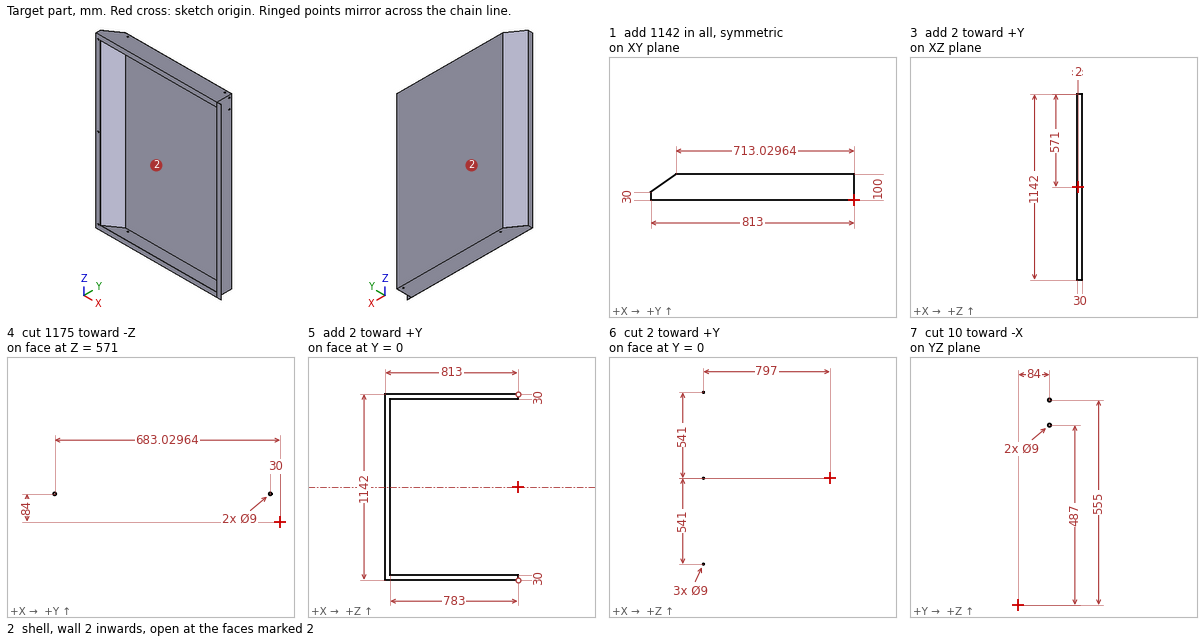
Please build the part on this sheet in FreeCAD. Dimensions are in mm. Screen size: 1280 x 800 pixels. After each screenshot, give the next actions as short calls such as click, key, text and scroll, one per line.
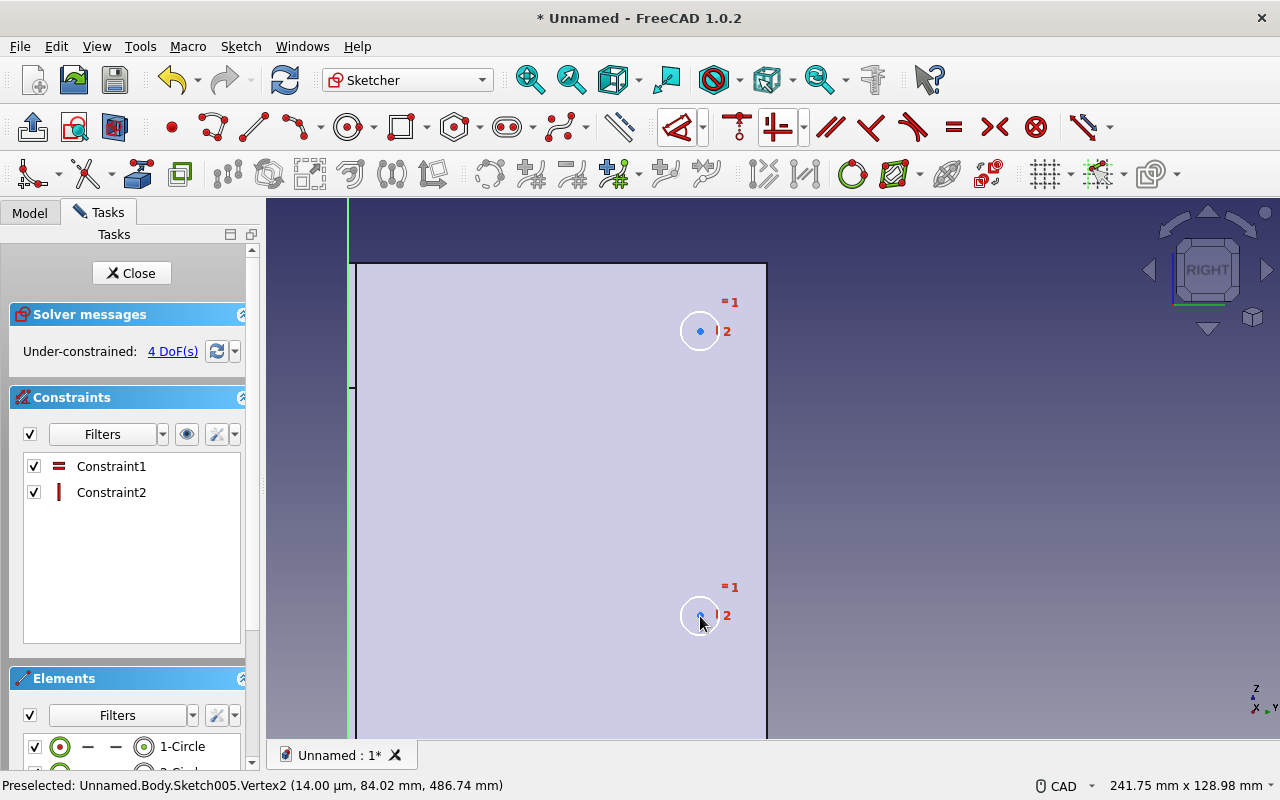
click(713, 317)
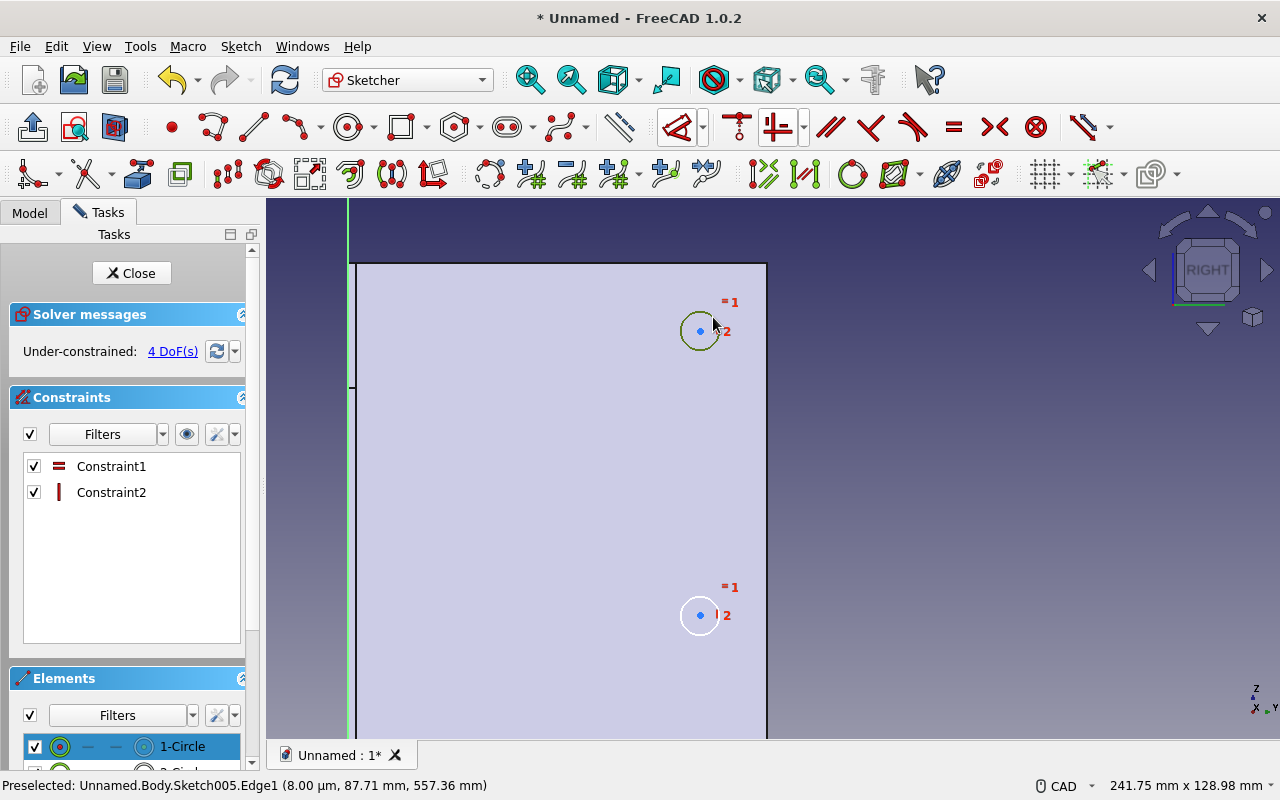
click(702, 128)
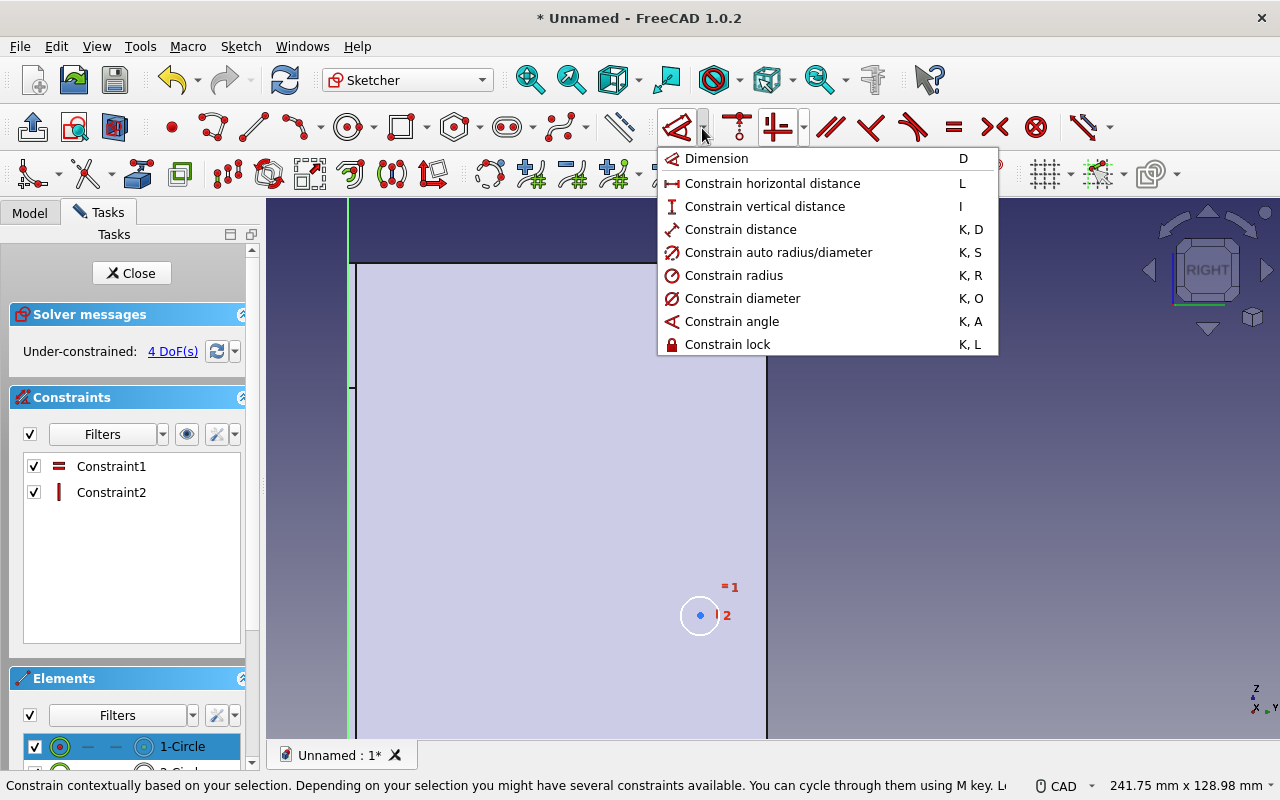
click(828, 298)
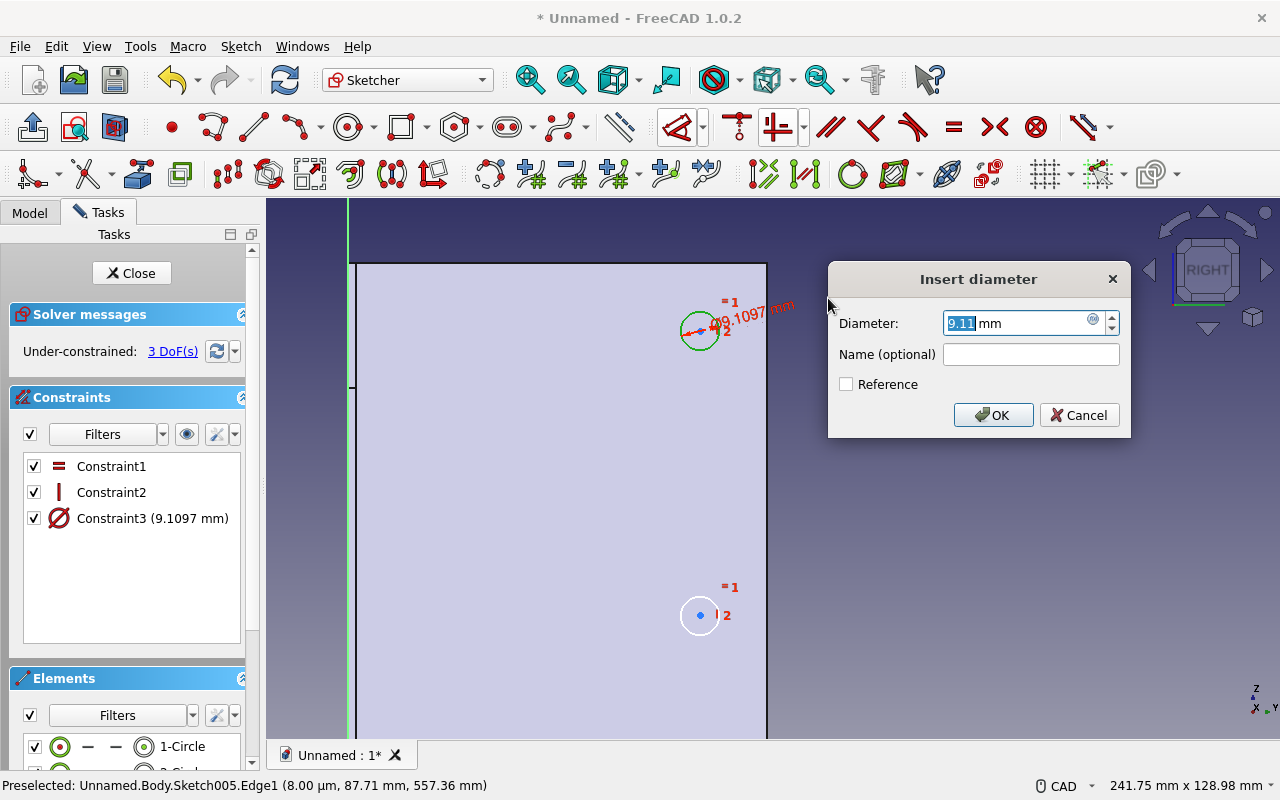
text(9)
key(Return)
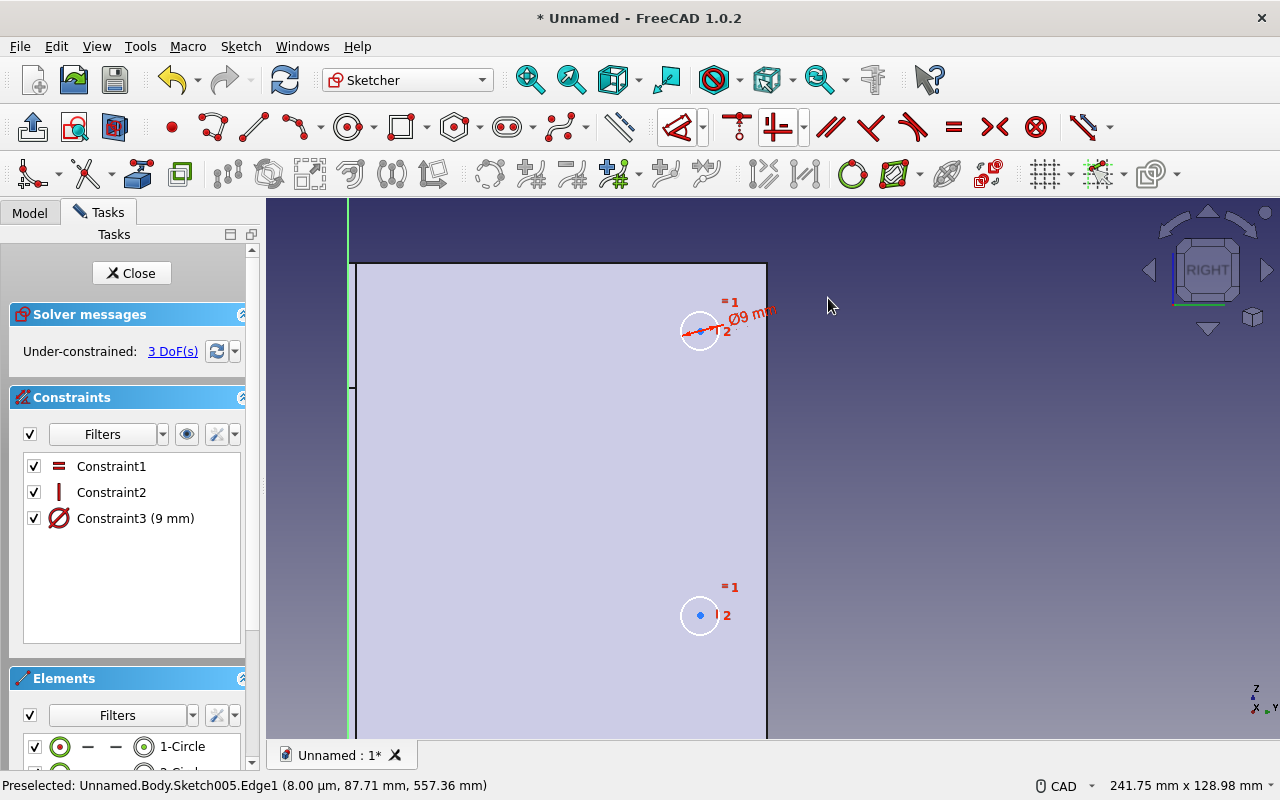
click(700, 331)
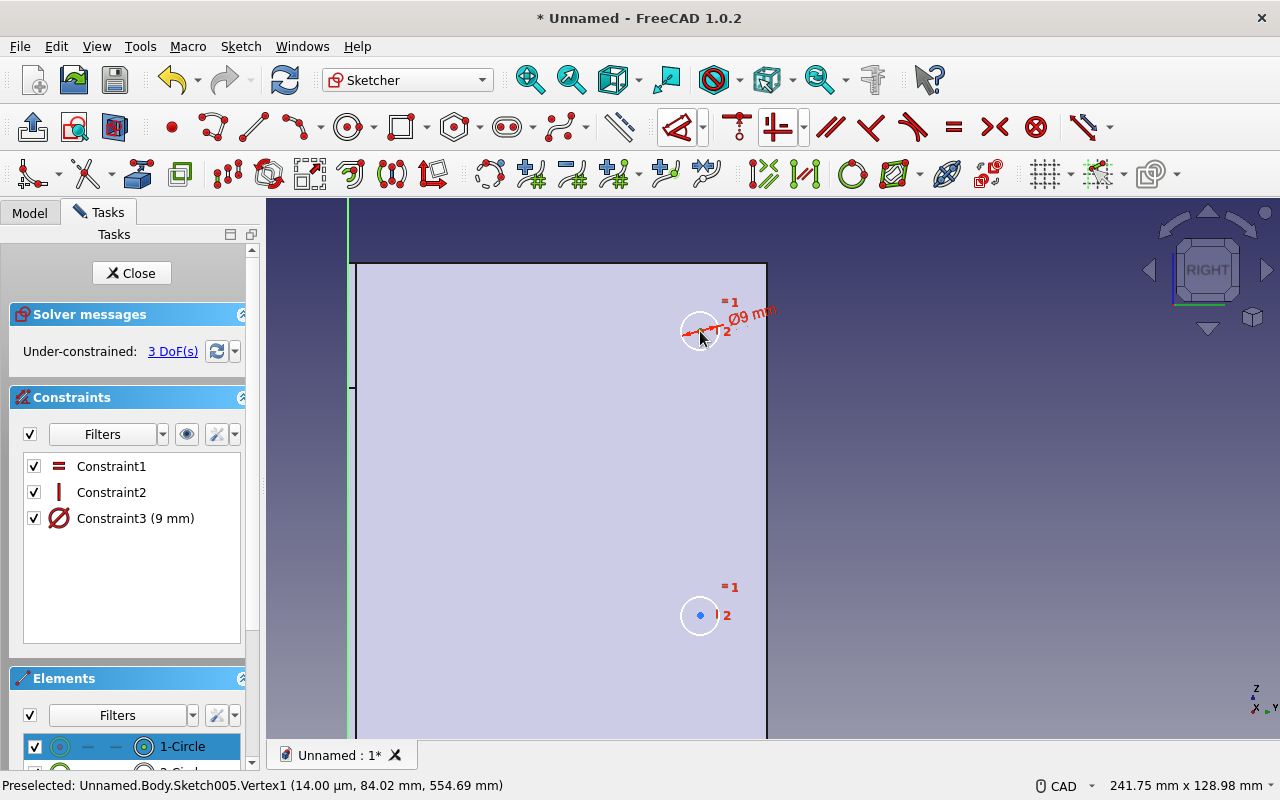
key(l)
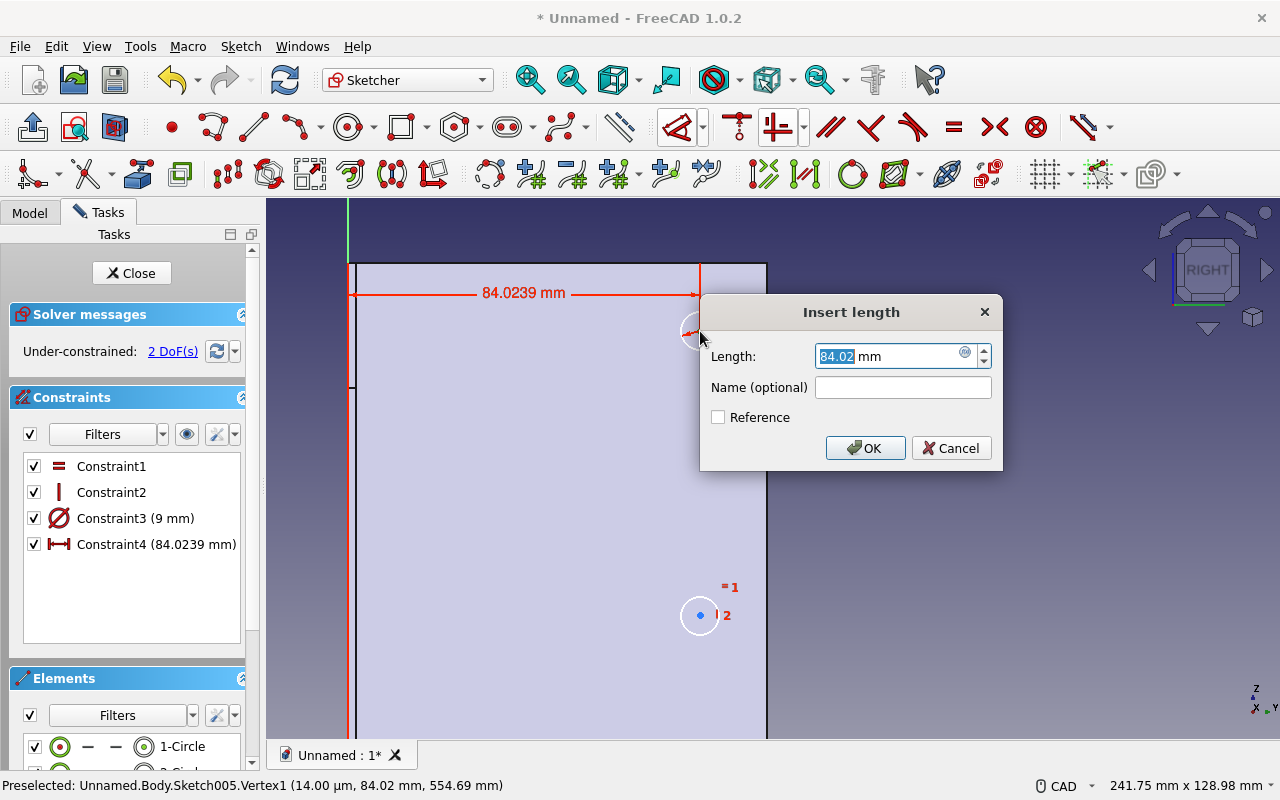
text(84)
key(Return)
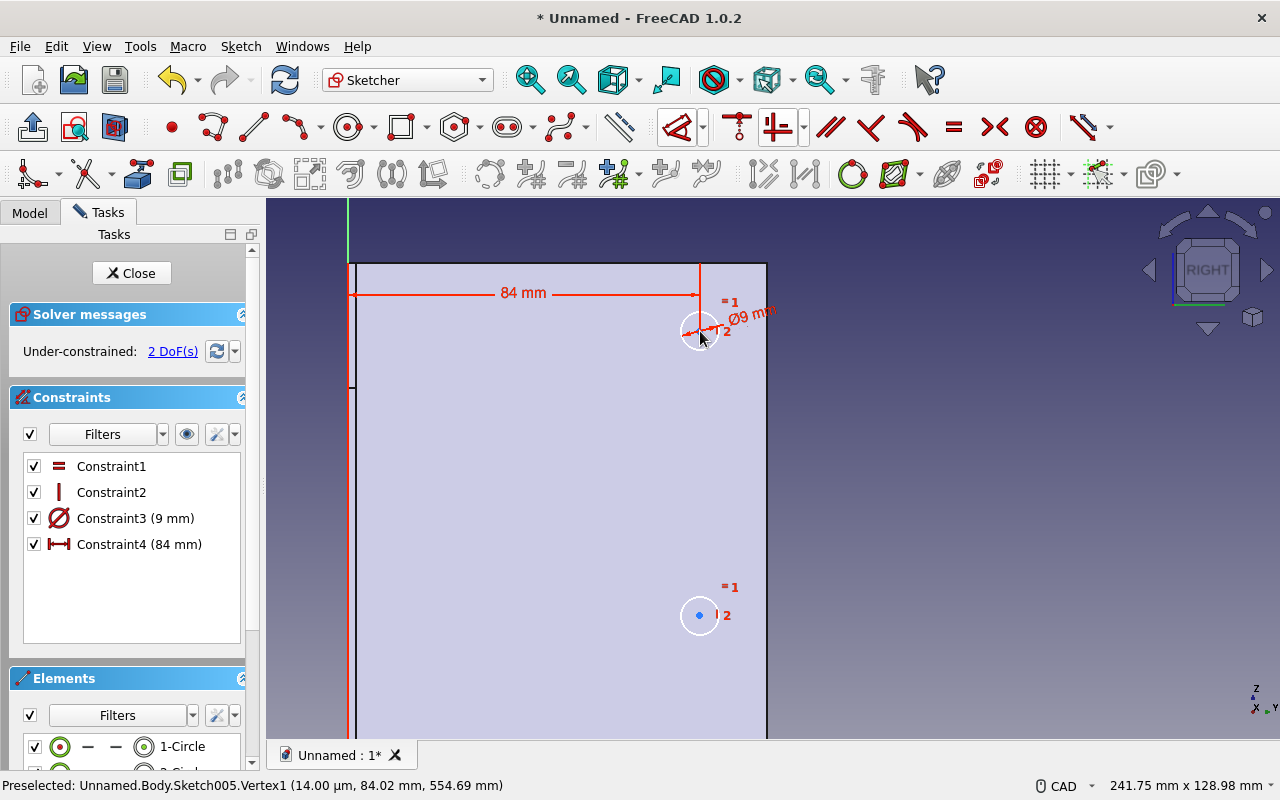
click(700, 331)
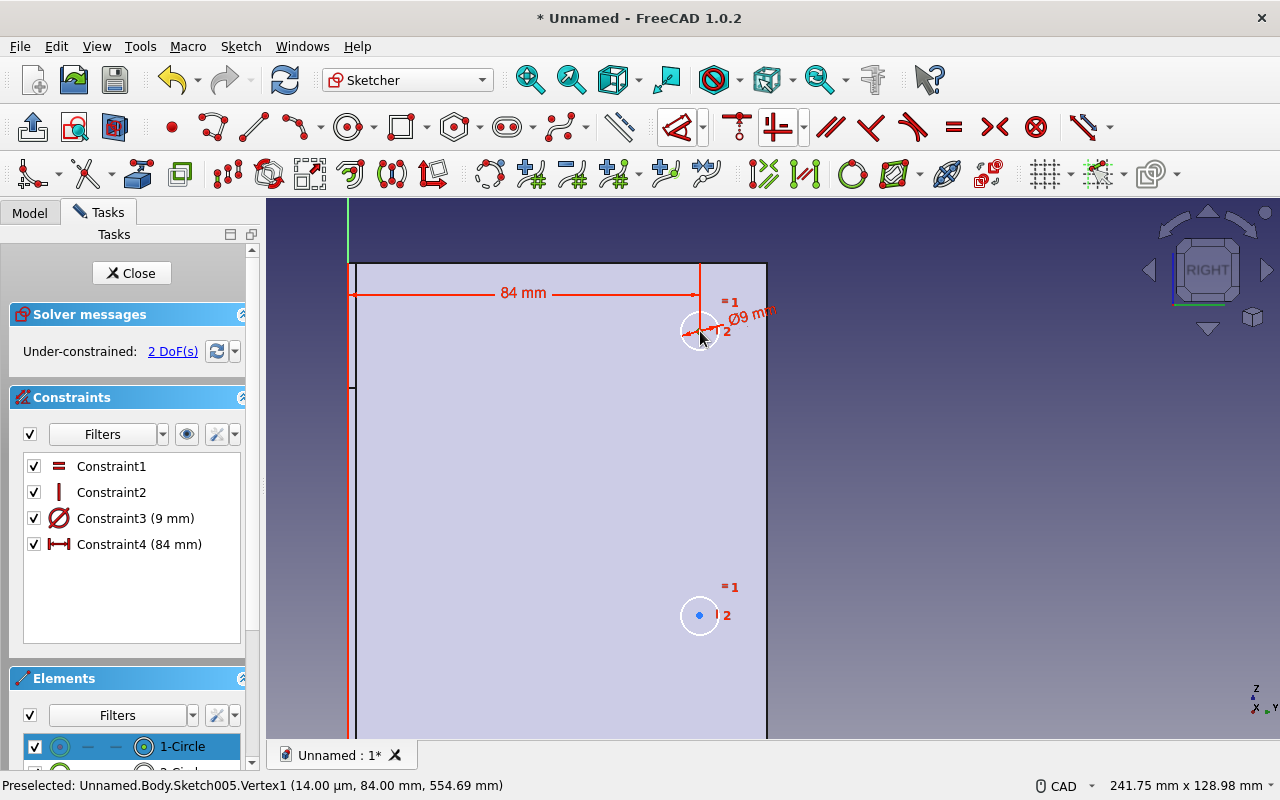
click(702, 128)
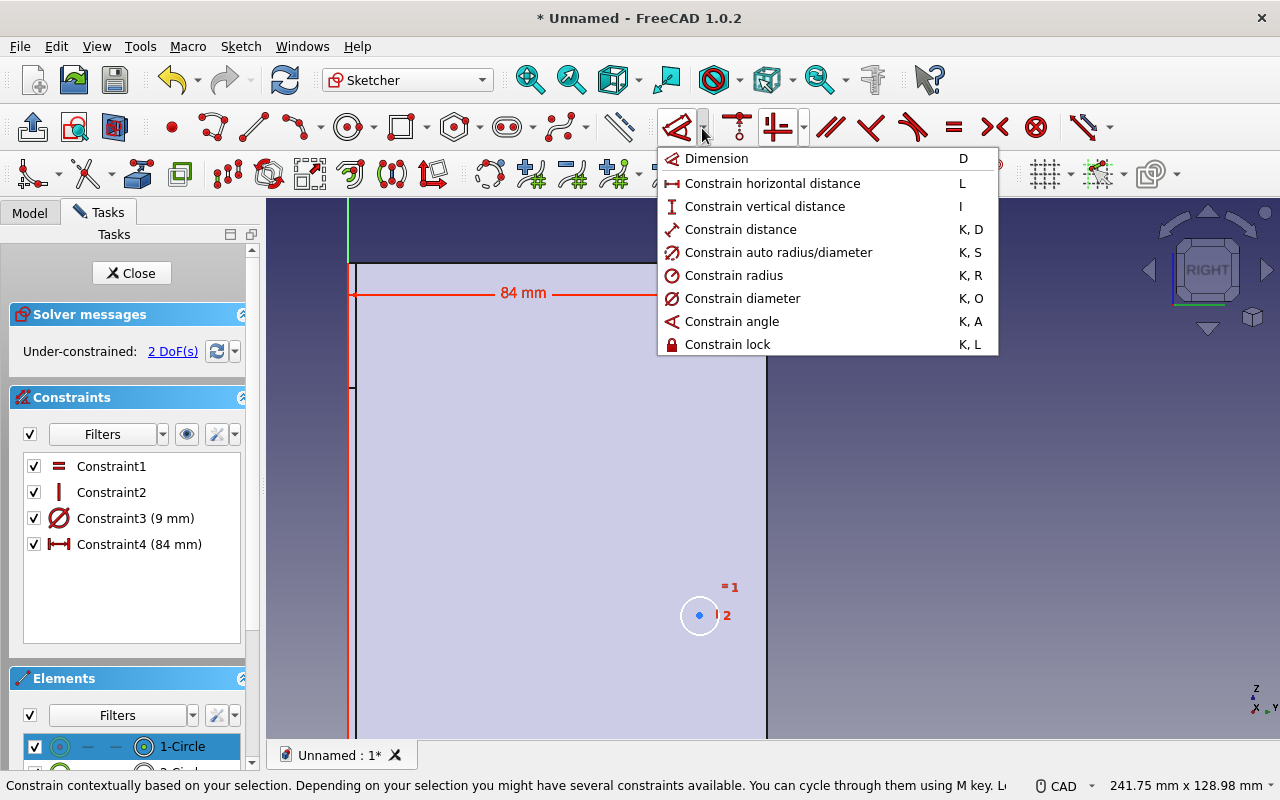
click(828, 206)